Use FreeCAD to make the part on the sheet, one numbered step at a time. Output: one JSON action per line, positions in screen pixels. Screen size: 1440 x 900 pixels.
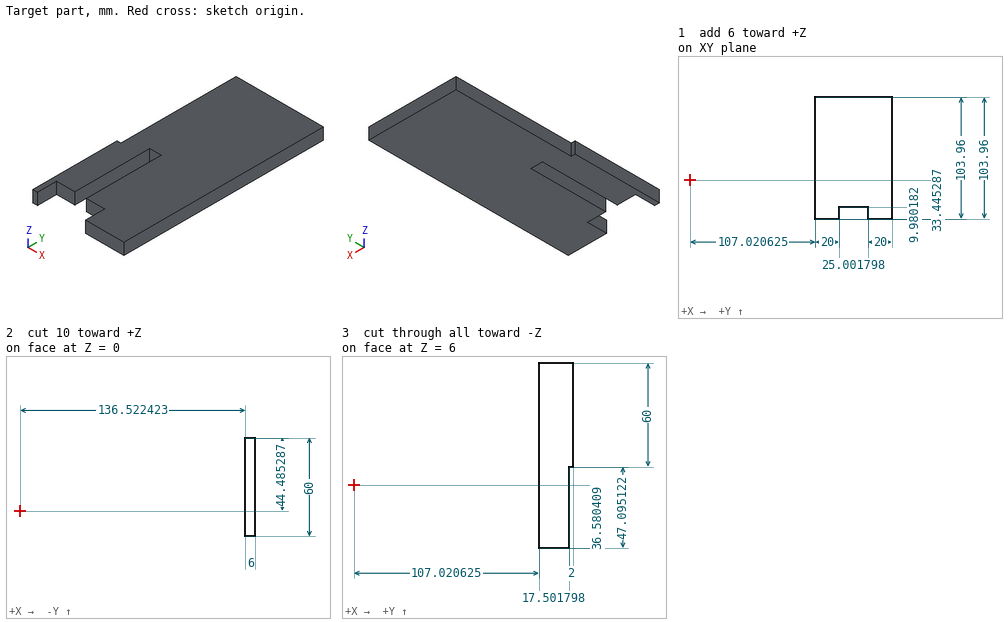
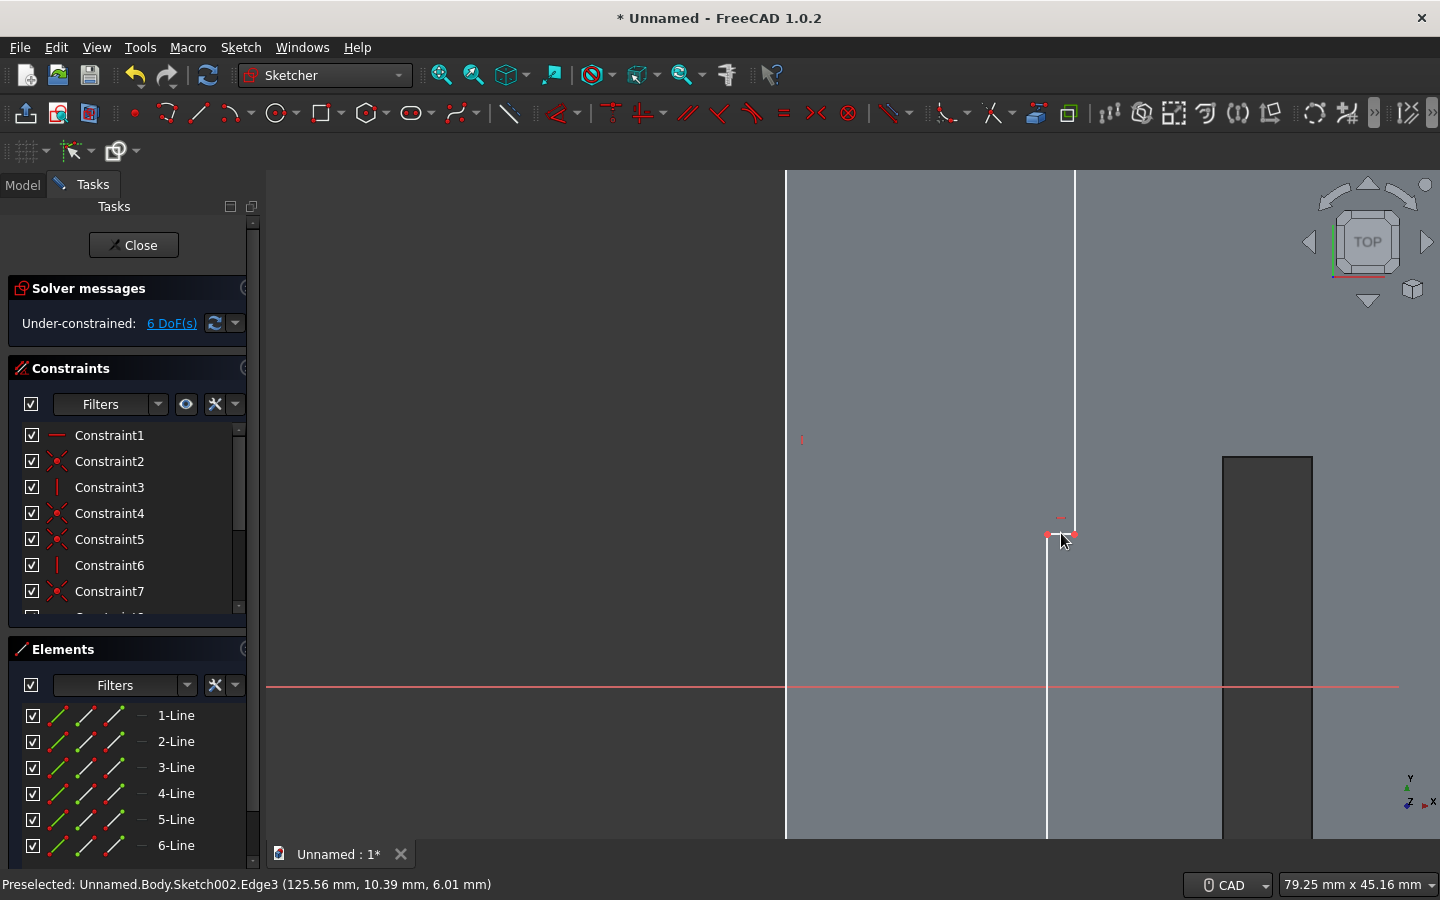
{"action": "left_click", "coordinate": [556, 114]}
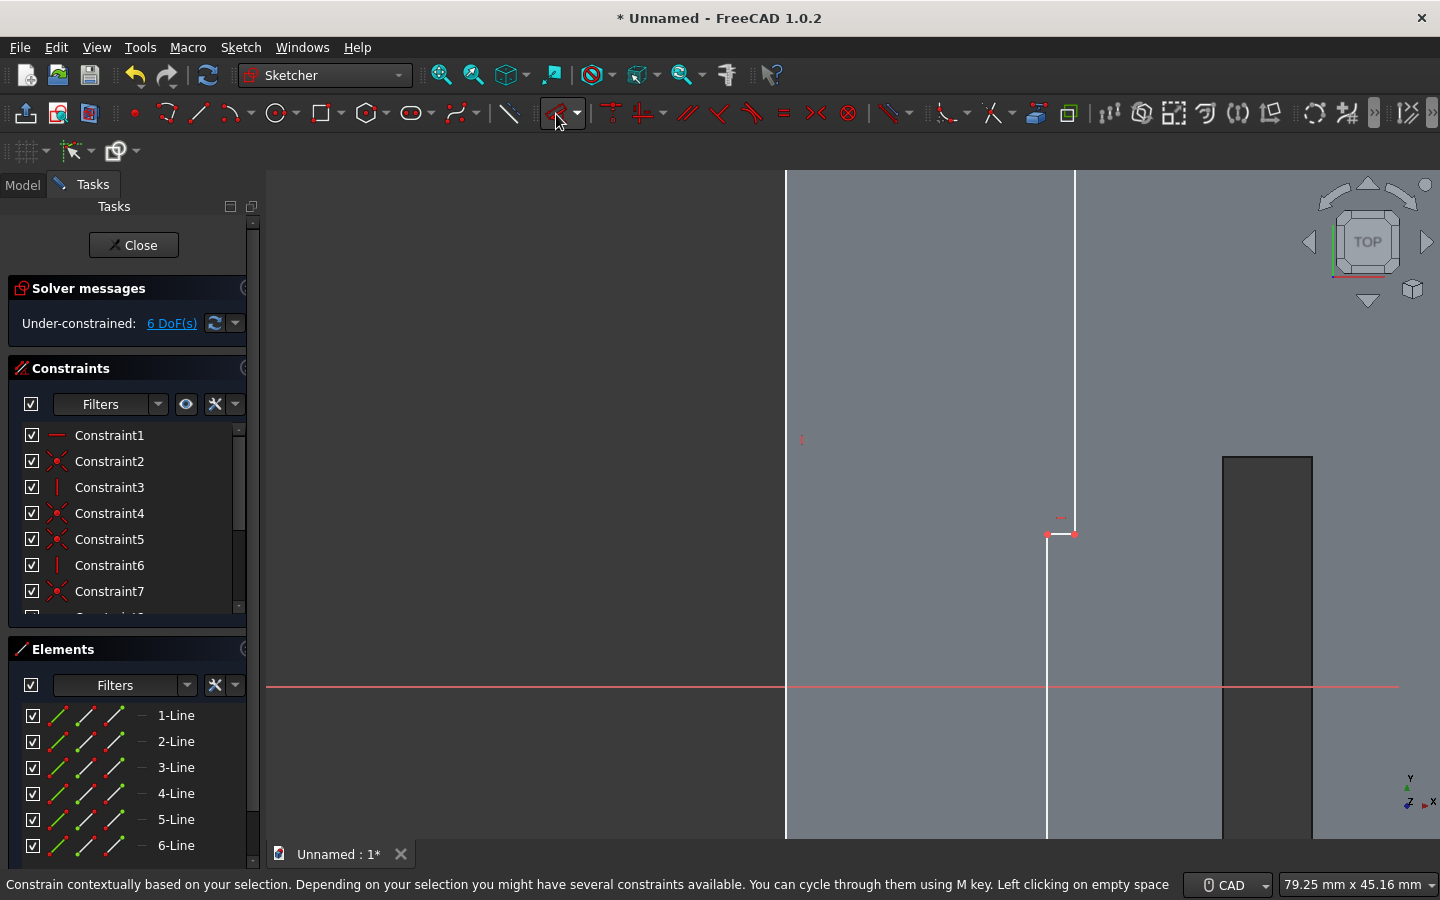
{"action": "scroll", "coordinate": [1058, 534], "scroll_direction": "up", "scroll_amount": 2}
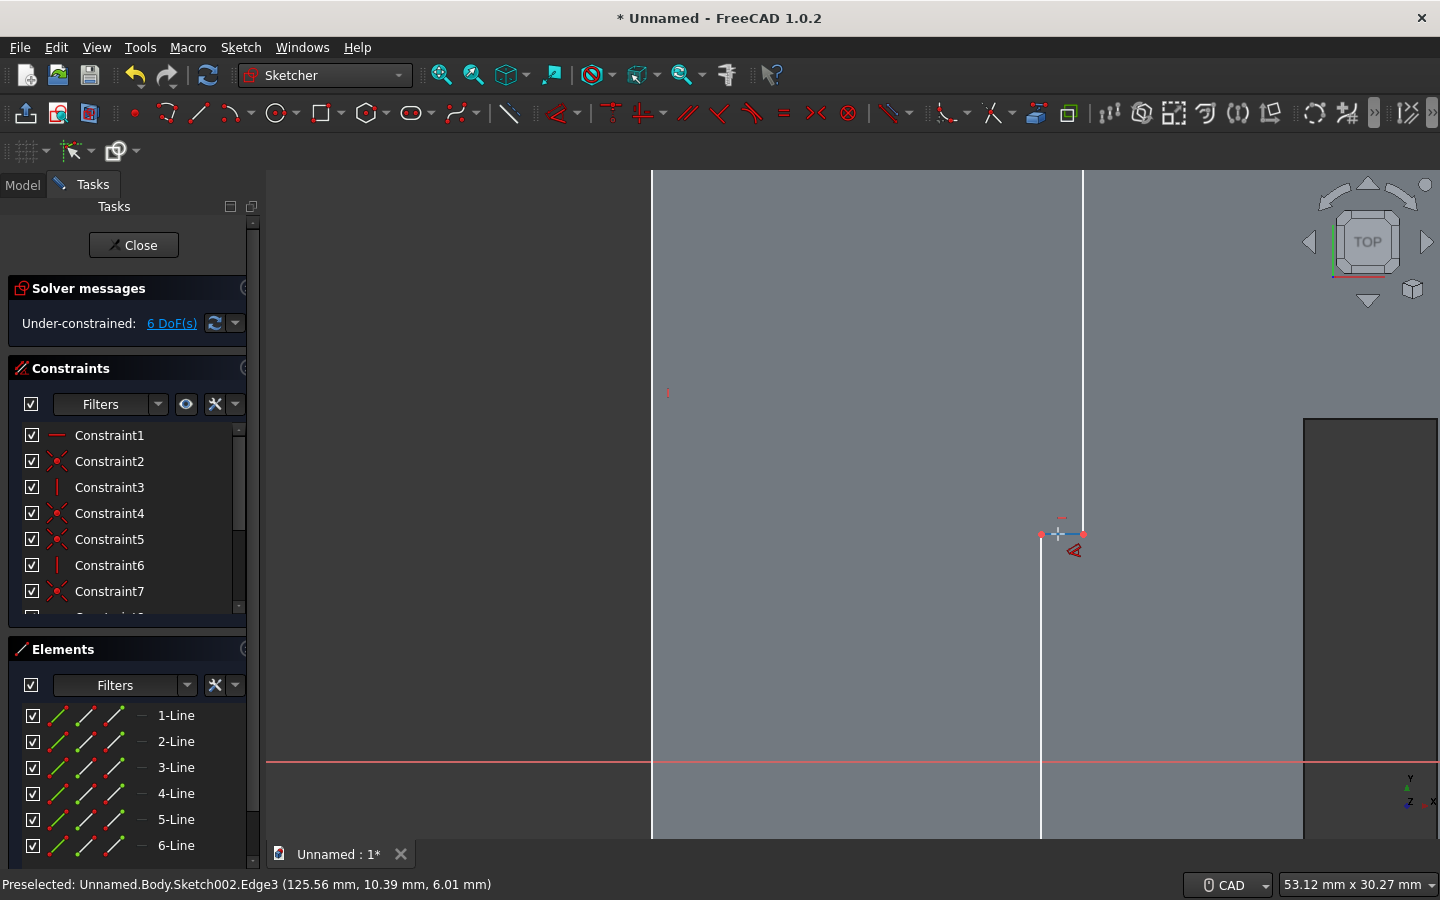
{"action": "left_click", "coordinate": [1058, 534]}
{"action": "left_click", "coordinate": [1062, 568]}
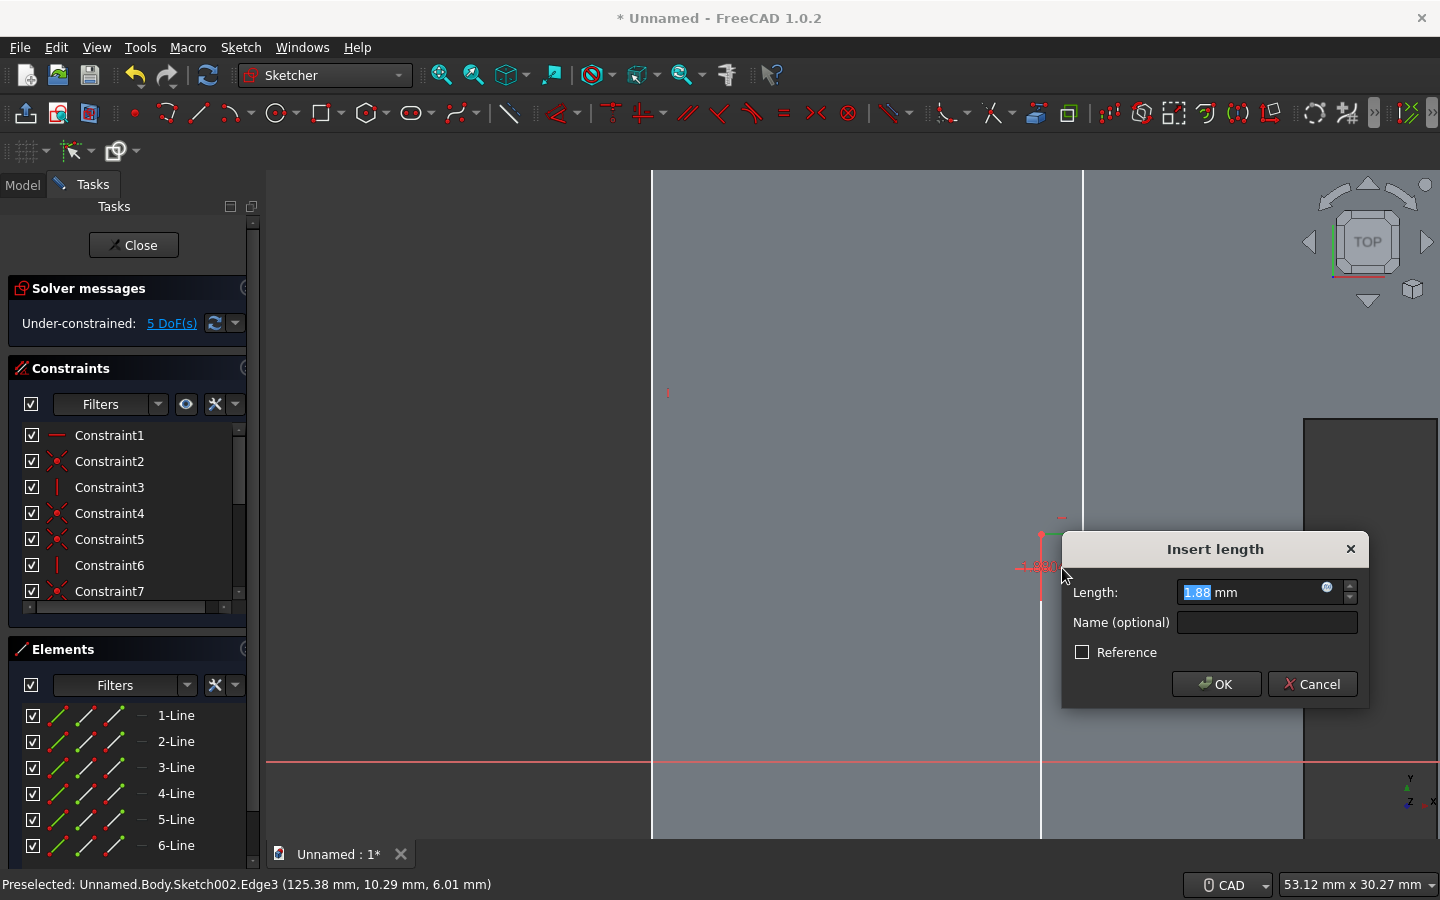
{"action": "type", "text": "2"}
{"action": "key", "text": "Return"}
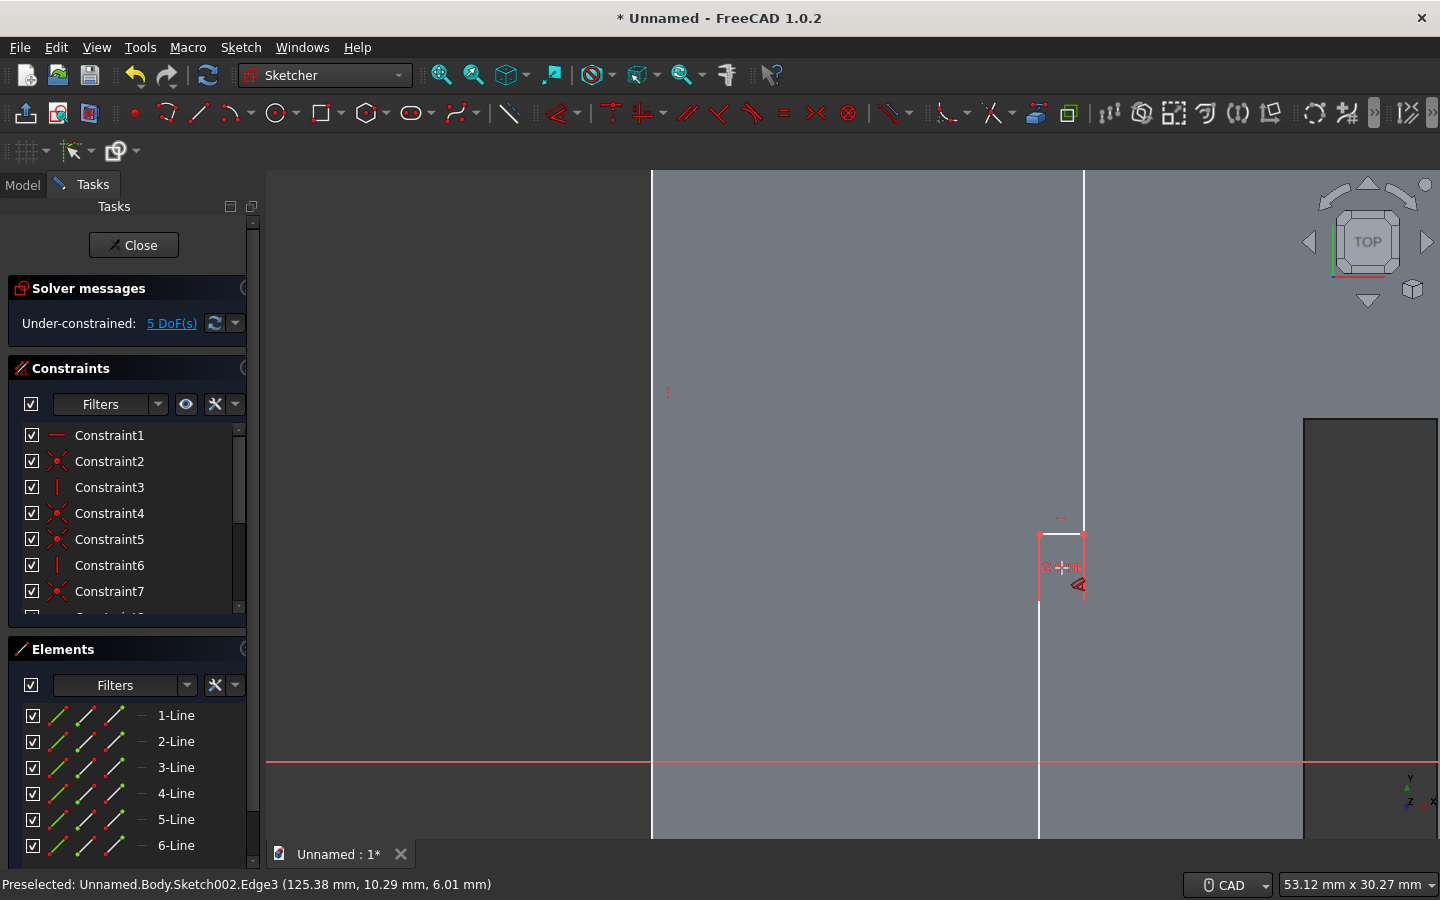
{"action": "scroll", "coordinate": [1063, 534], "scroll_direction": "down", "scroll_amount": 8}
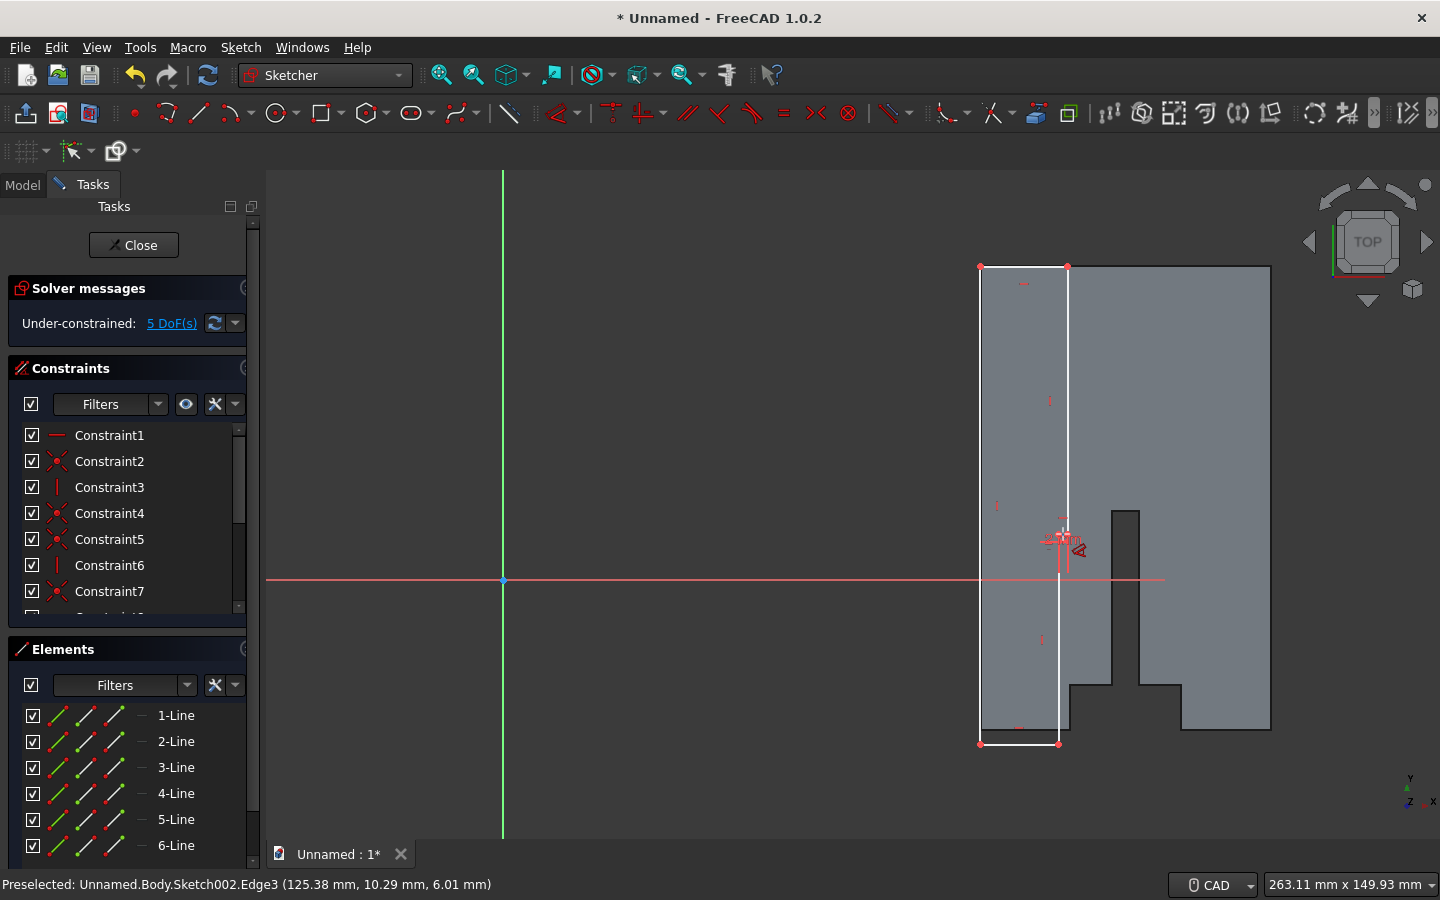
{"action": "left_click", "coordinate": [1068, 481]}
{"action": "left_click", "coordinate": [1102, 401]}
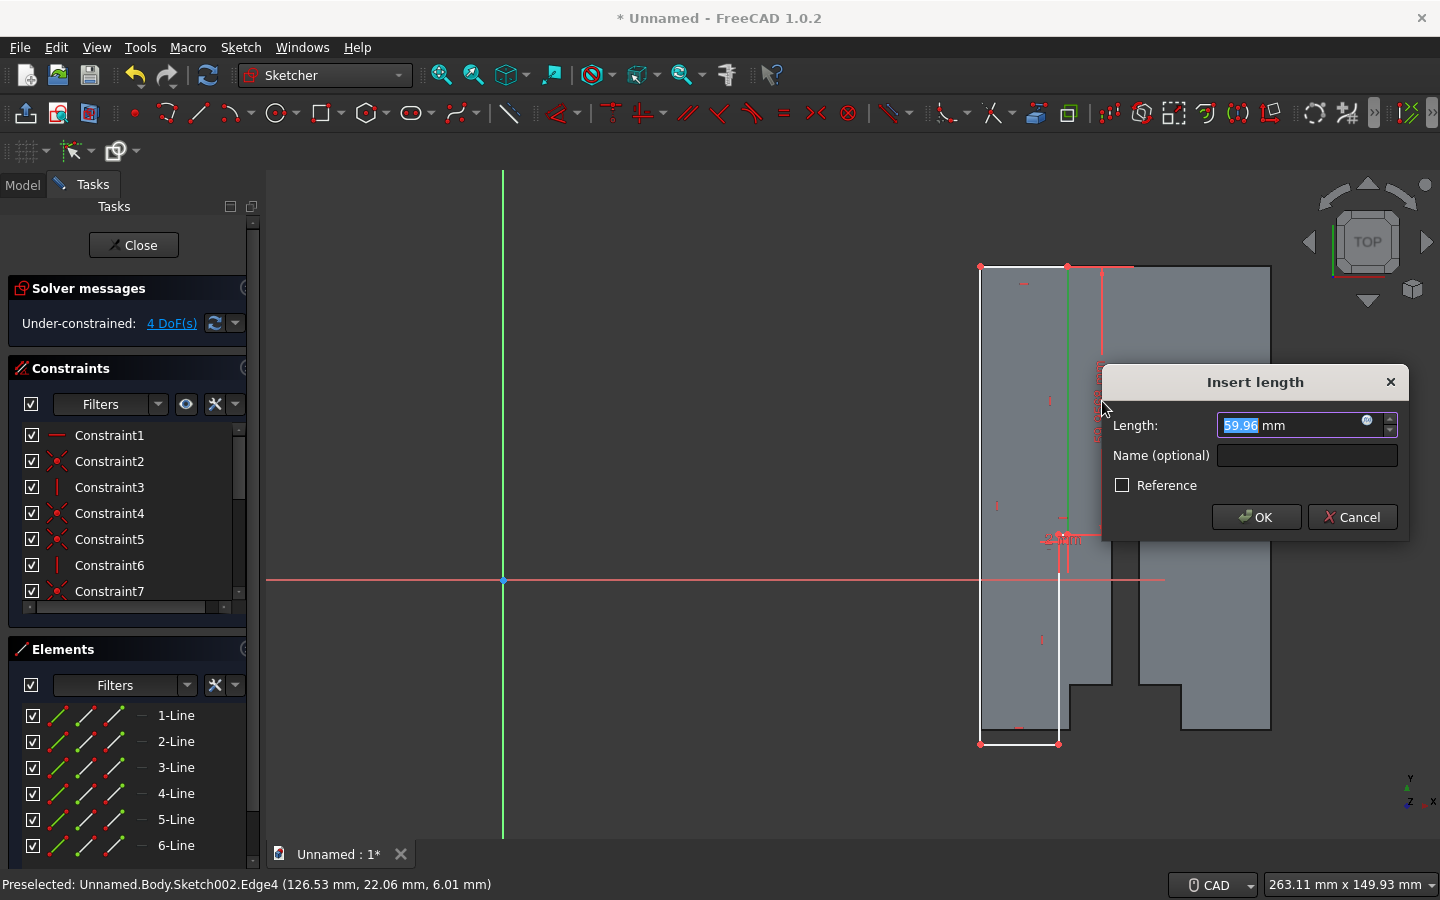
{"action": "type", "text": "60"}
{"action": "key", "text": "Return"}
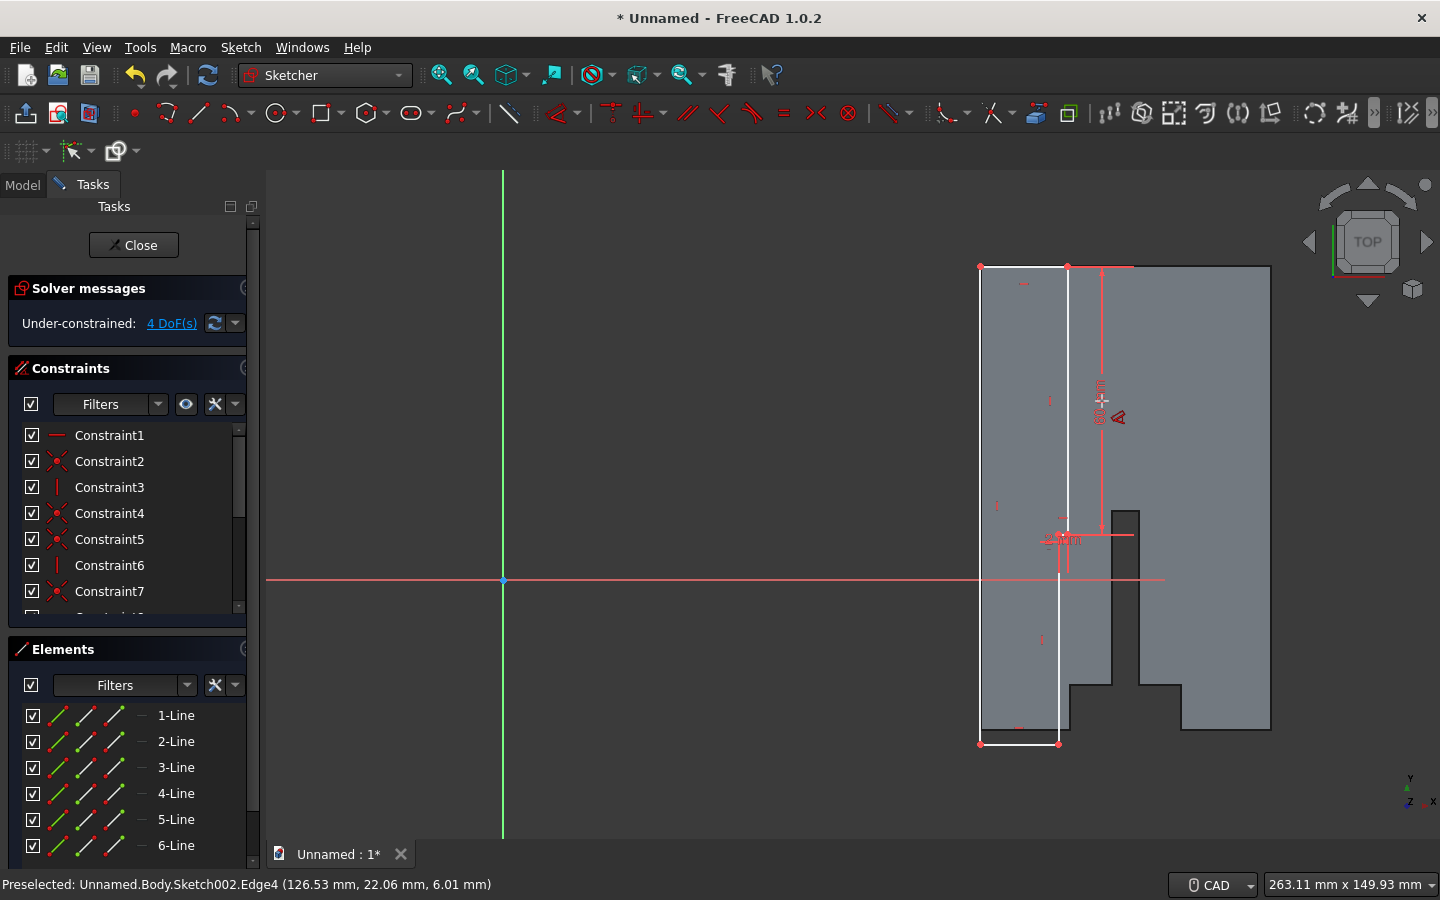
{"action": "left_click", "coordinate": [1004, 745]}
{"action": "left_click", "coordinate": [1020, 779]}